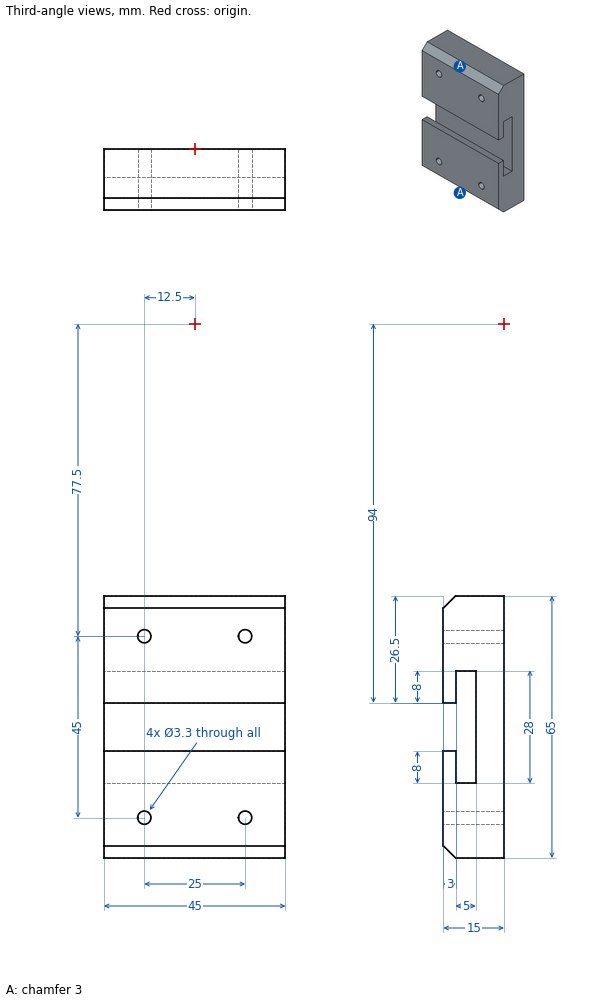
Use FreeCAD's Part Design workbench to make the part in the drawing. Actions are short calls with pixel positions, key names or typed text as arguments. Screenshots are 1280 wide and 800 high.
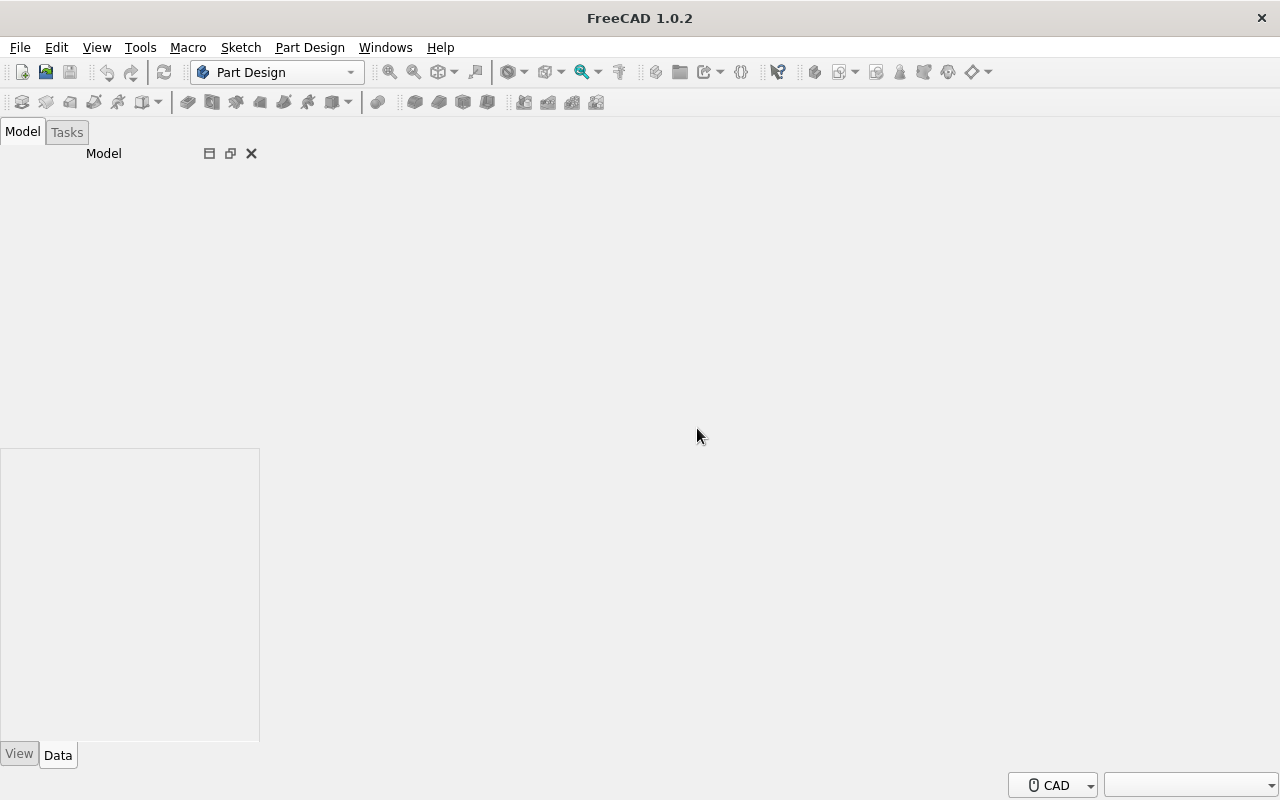
click(22, 72)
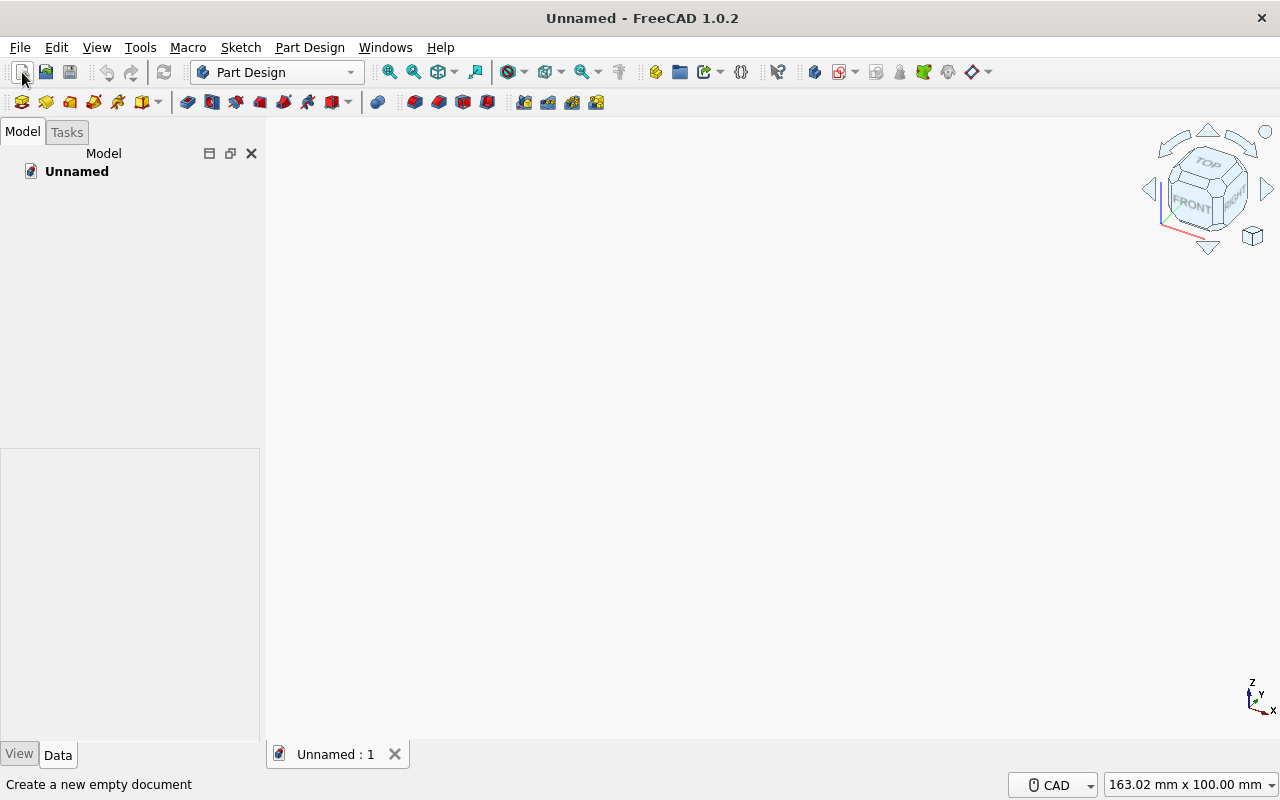
click(840, 72)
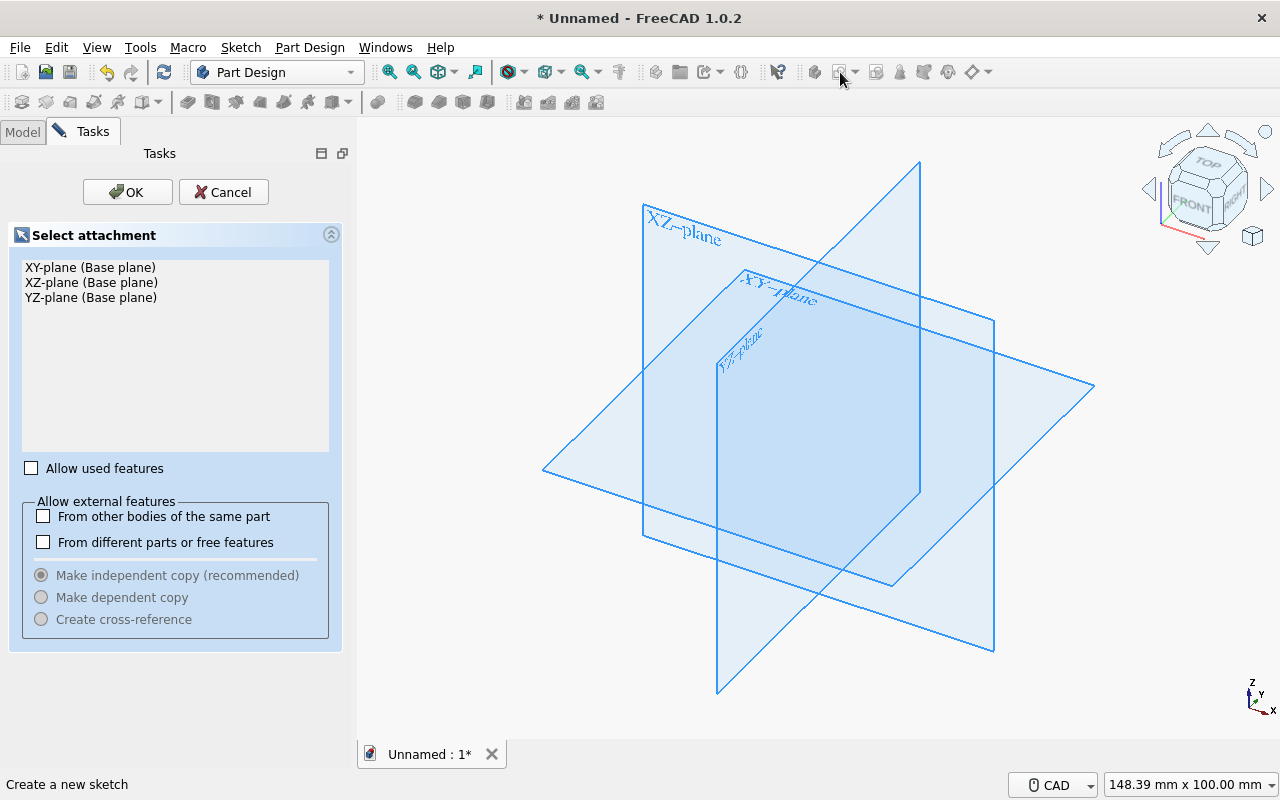
click(82, 298)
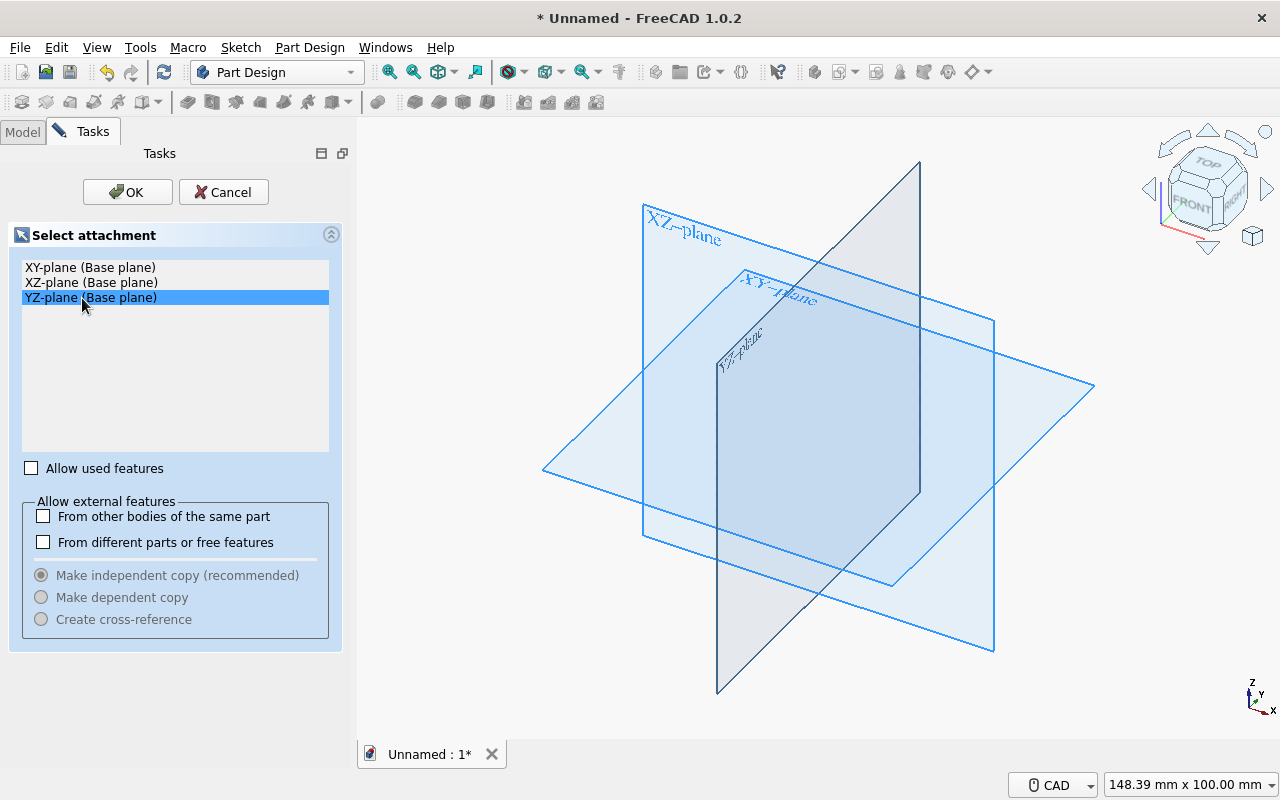
click(128, 192)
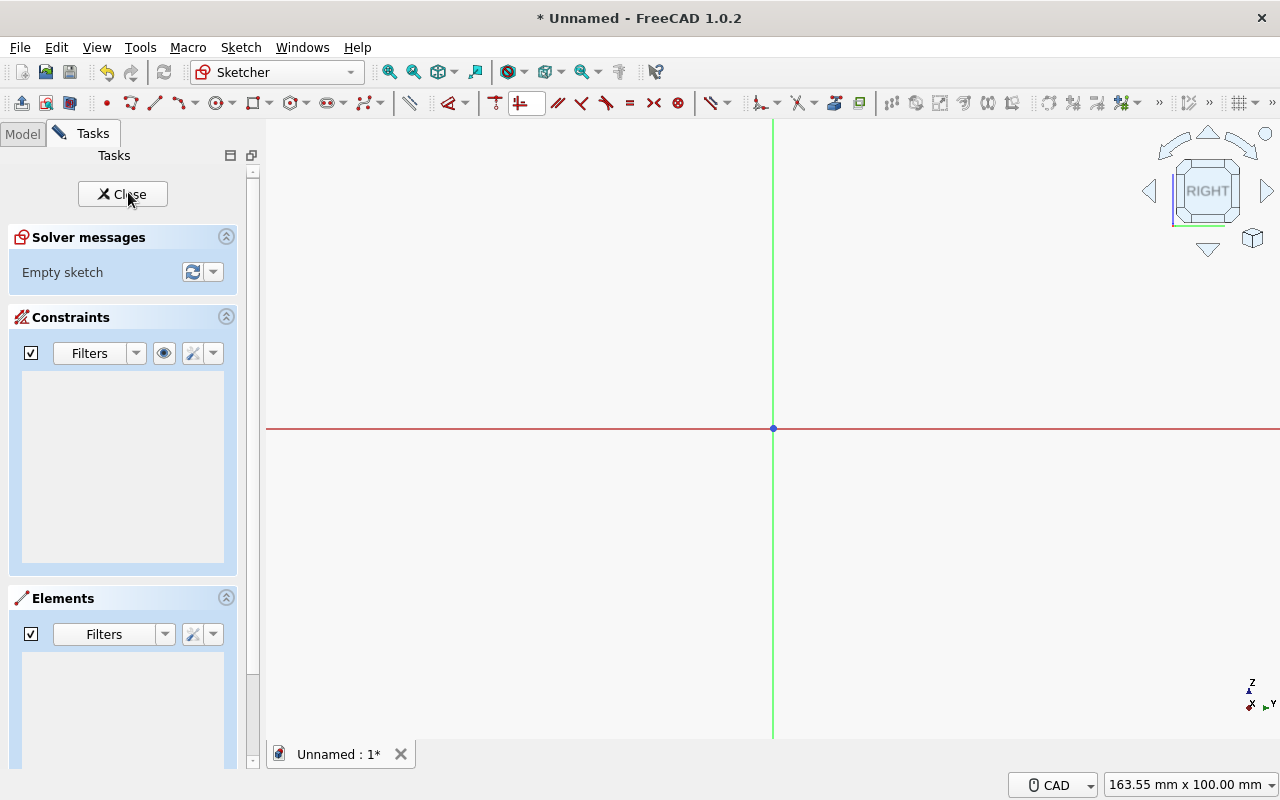
scroll(687, 147, down, 4)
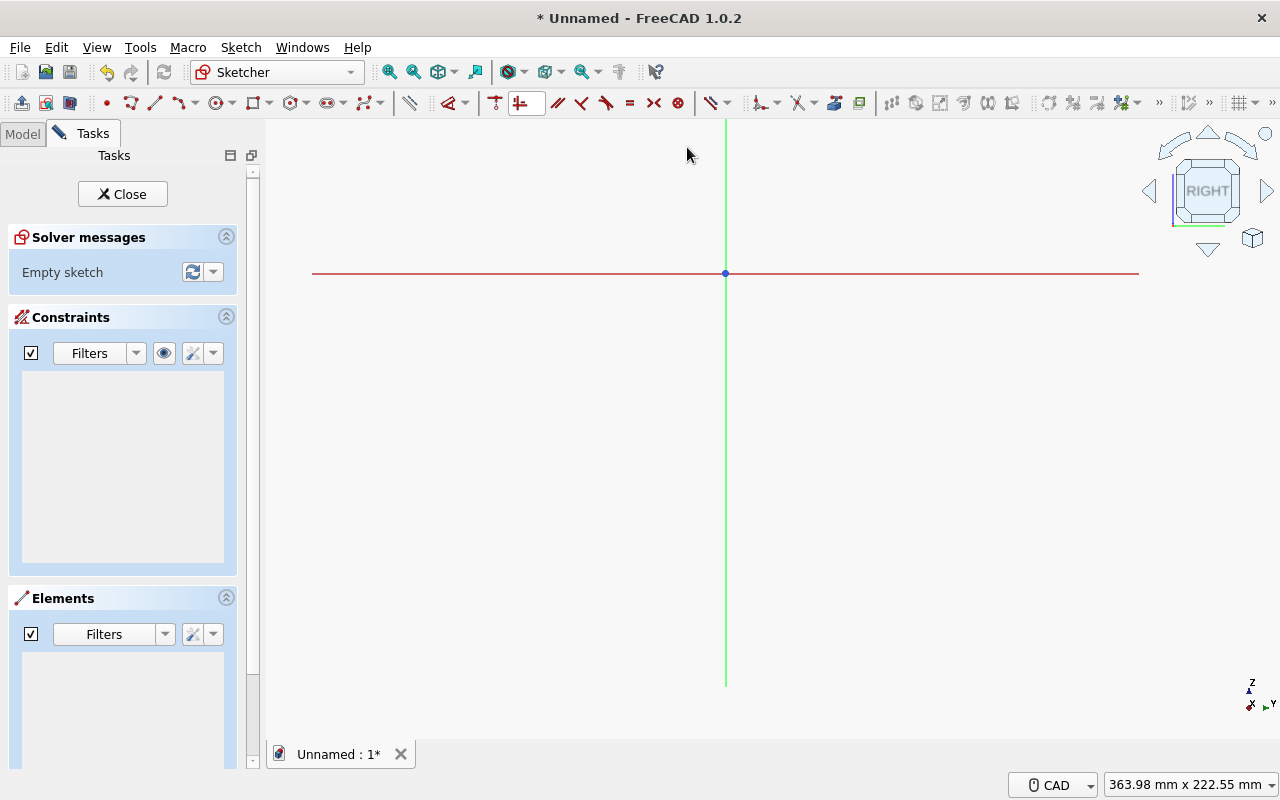
click(132, 104)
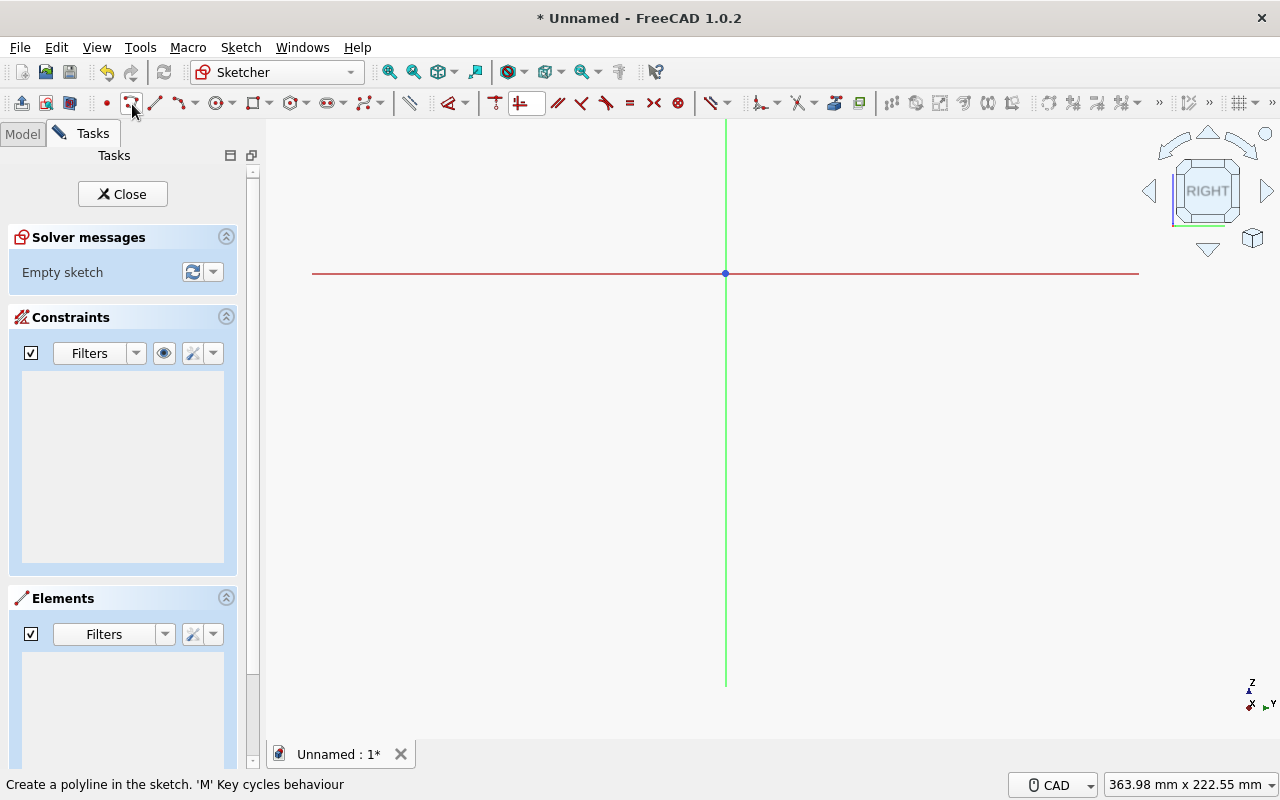
click(726, 462)
click(684, 462)
click(684, 536)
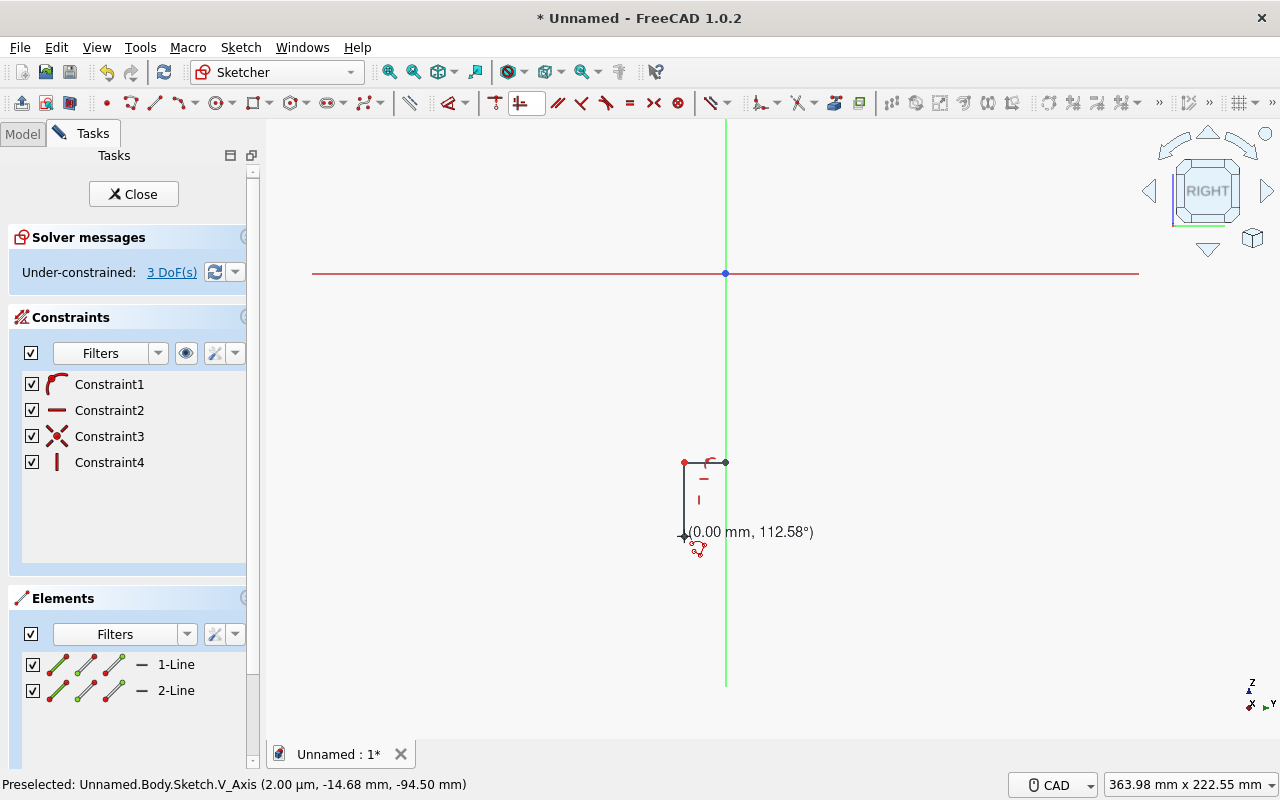
scroll(692, 536, up, 4)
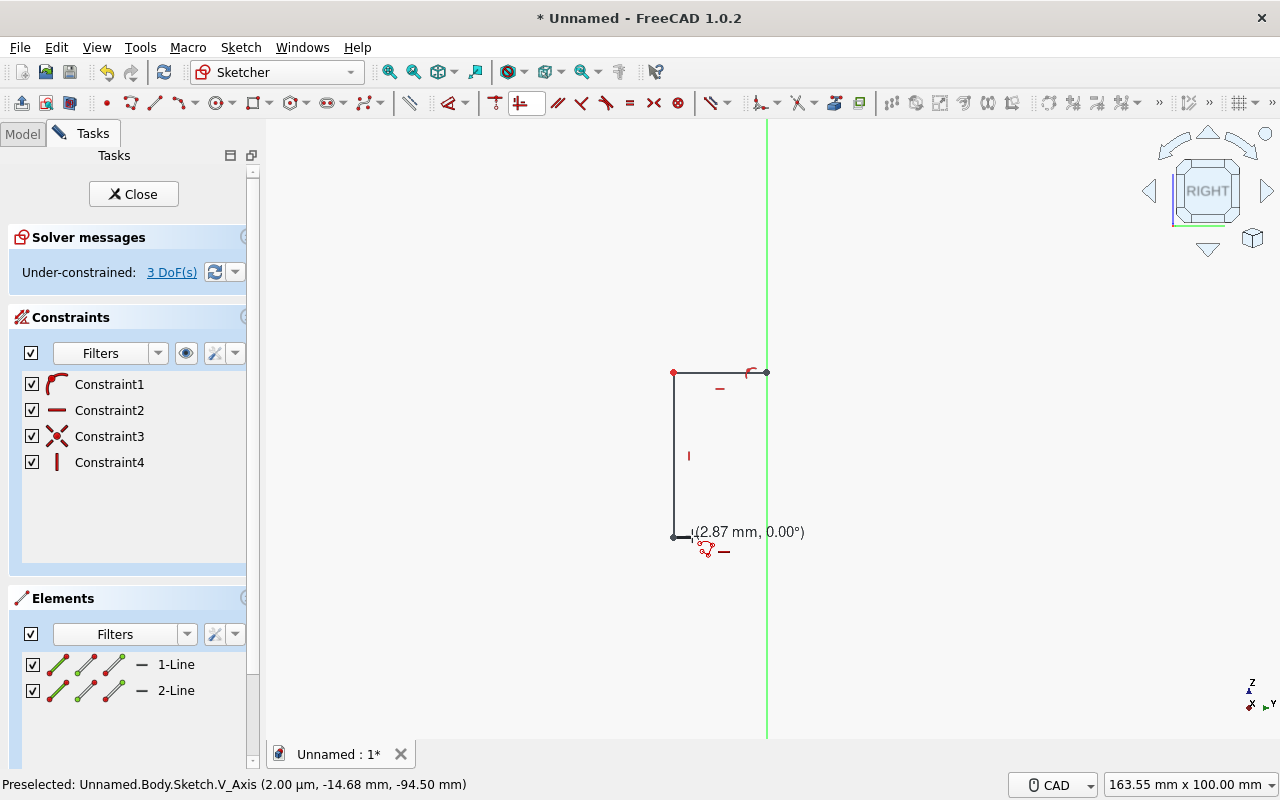
click(692, 535)
click(692, 485)
click(723, 485)
click(723, 658)
click(692, 658)
click(692, 609)
click(674, 609)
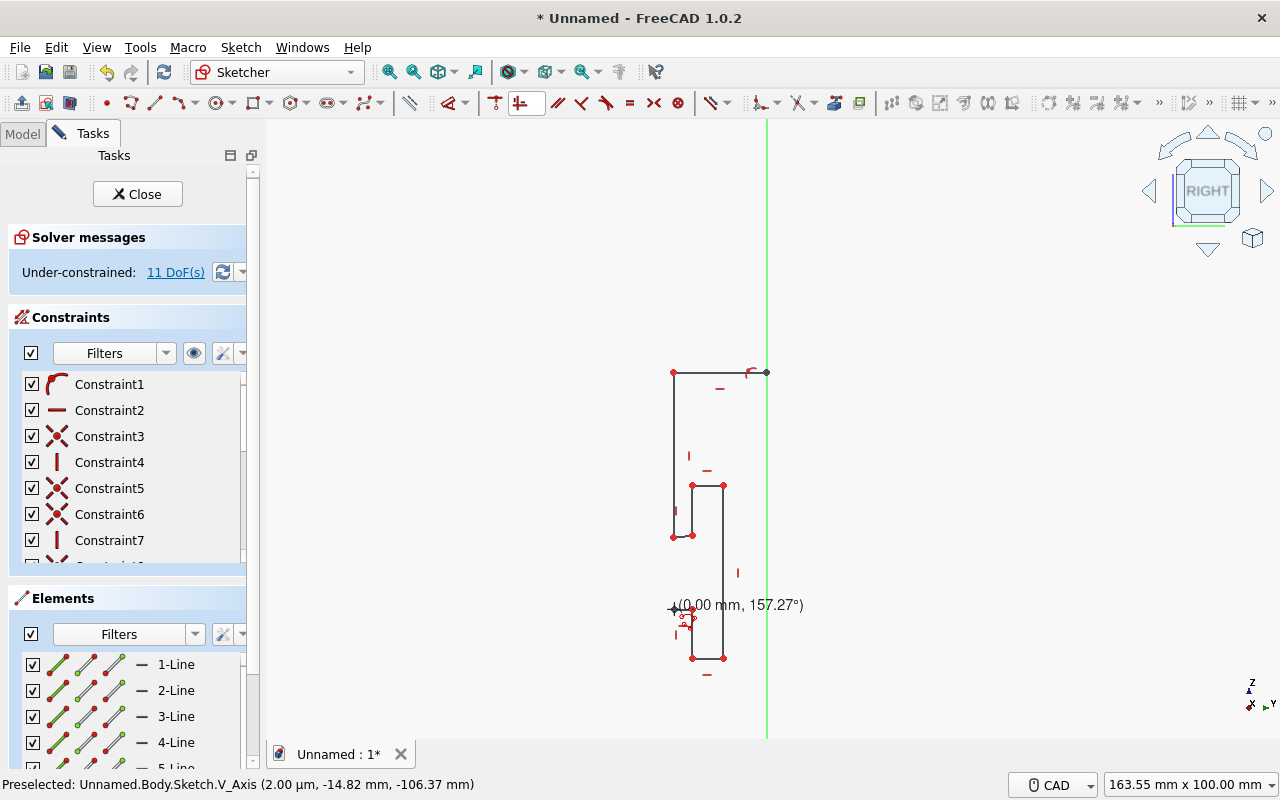
scroll(692, 483, down, 4)